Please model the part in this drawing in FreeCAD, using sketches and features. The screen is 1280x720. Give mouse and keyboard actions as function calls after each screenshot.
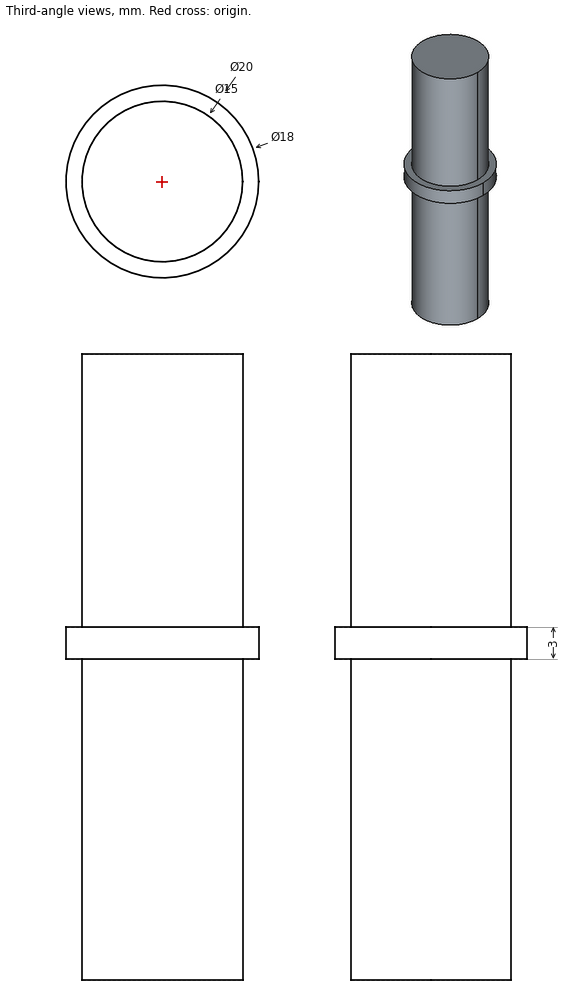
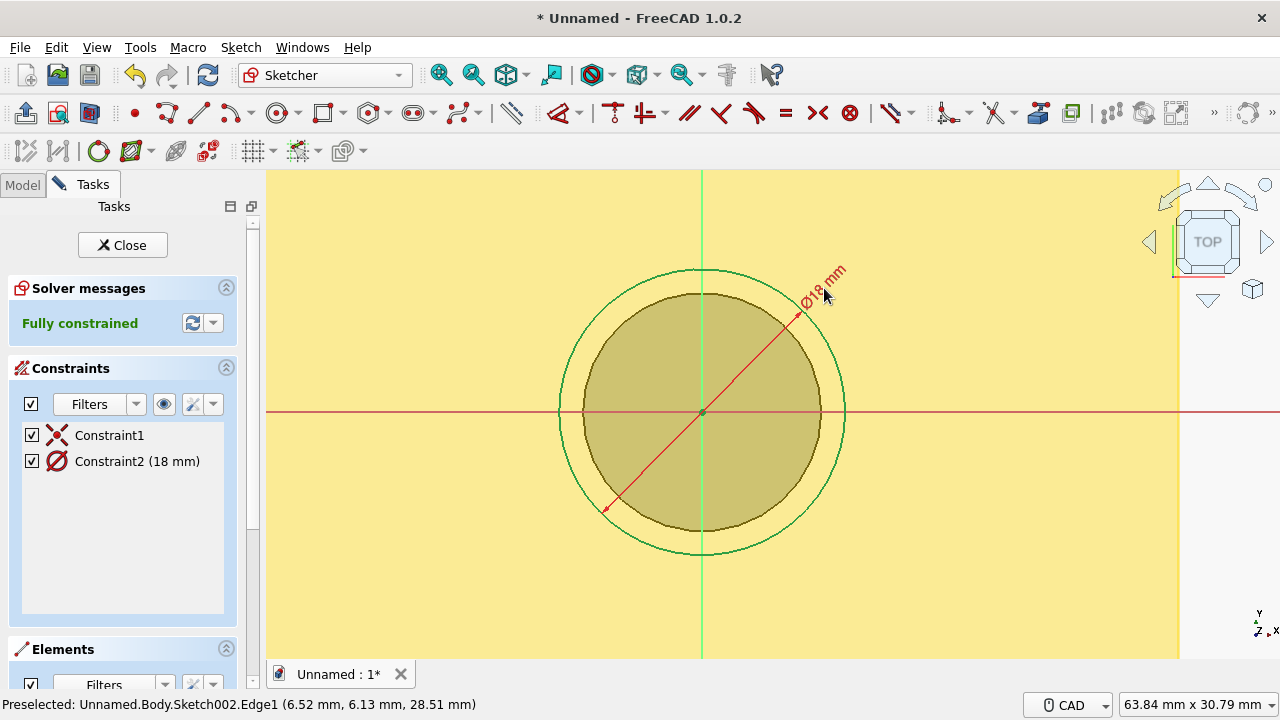
click(123, 245)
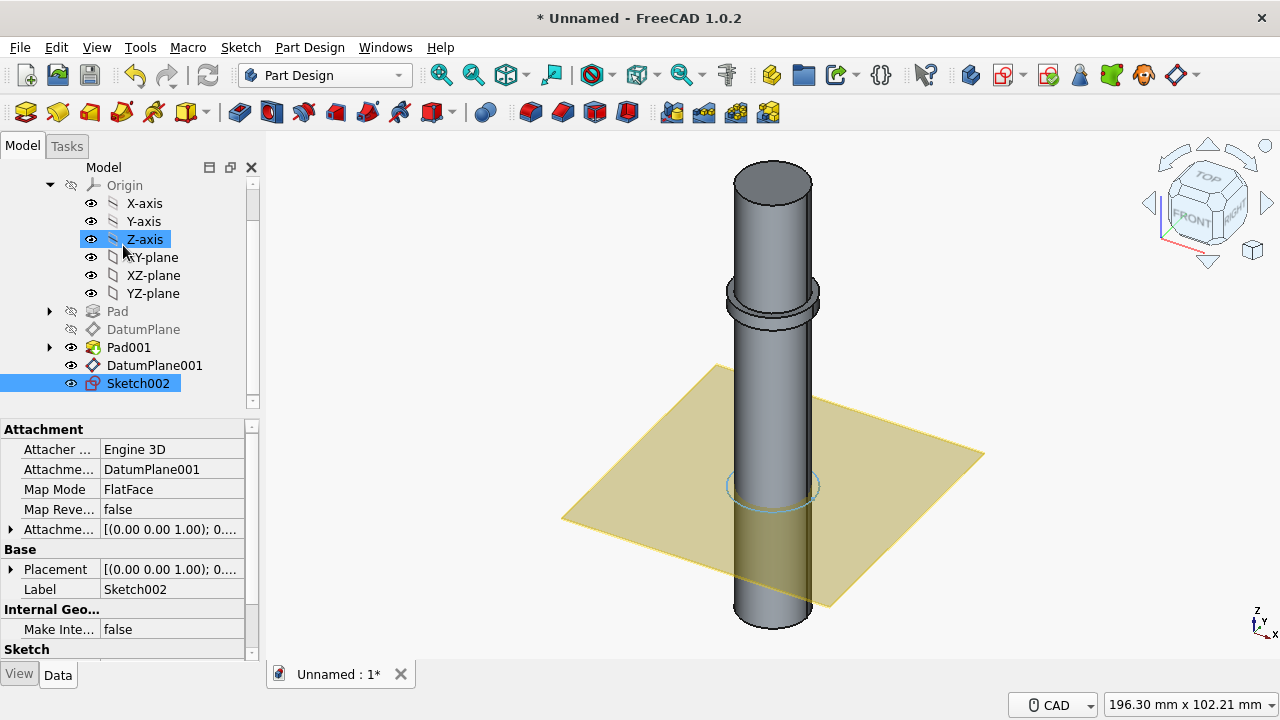
click(26, 112)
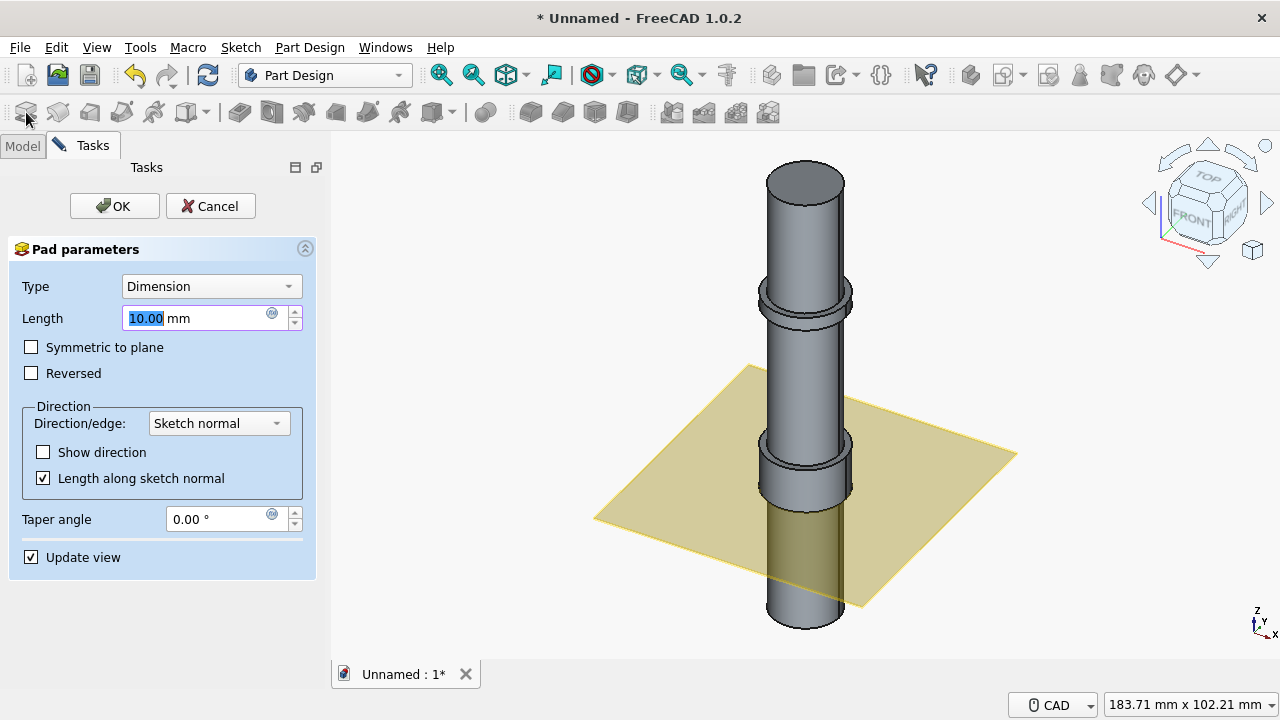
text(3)
key(Tab)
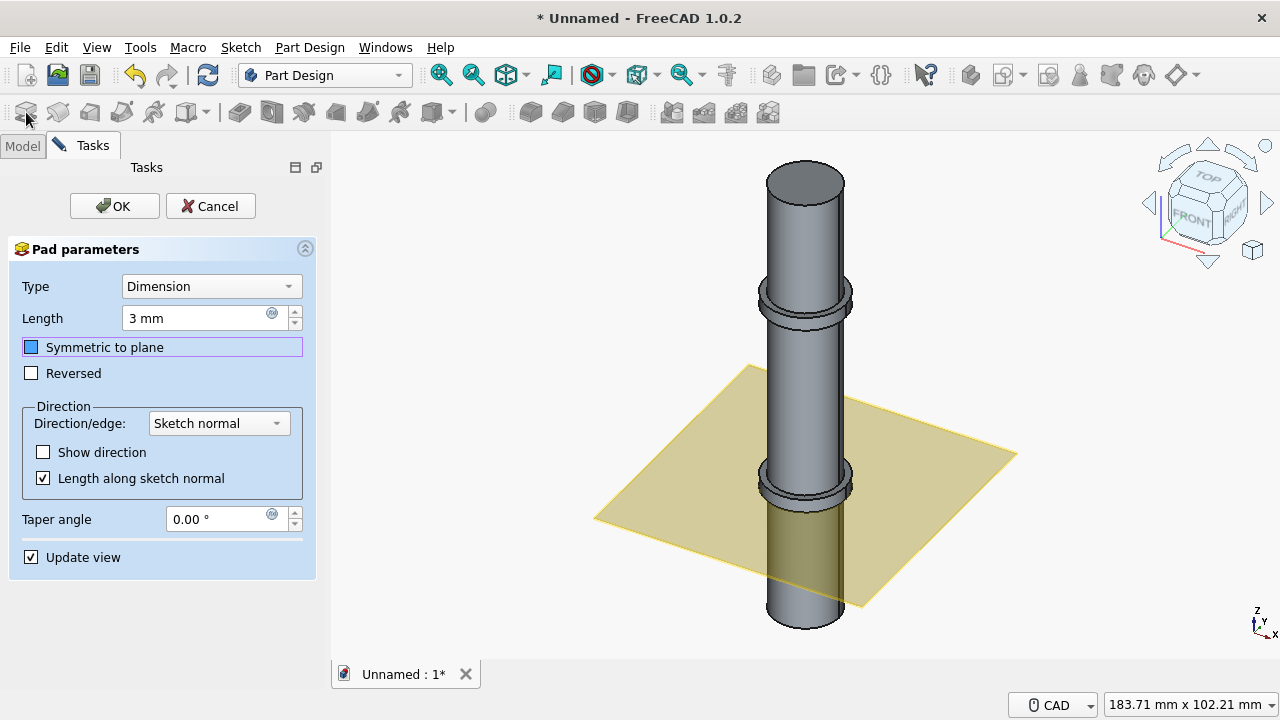
click(30, 373)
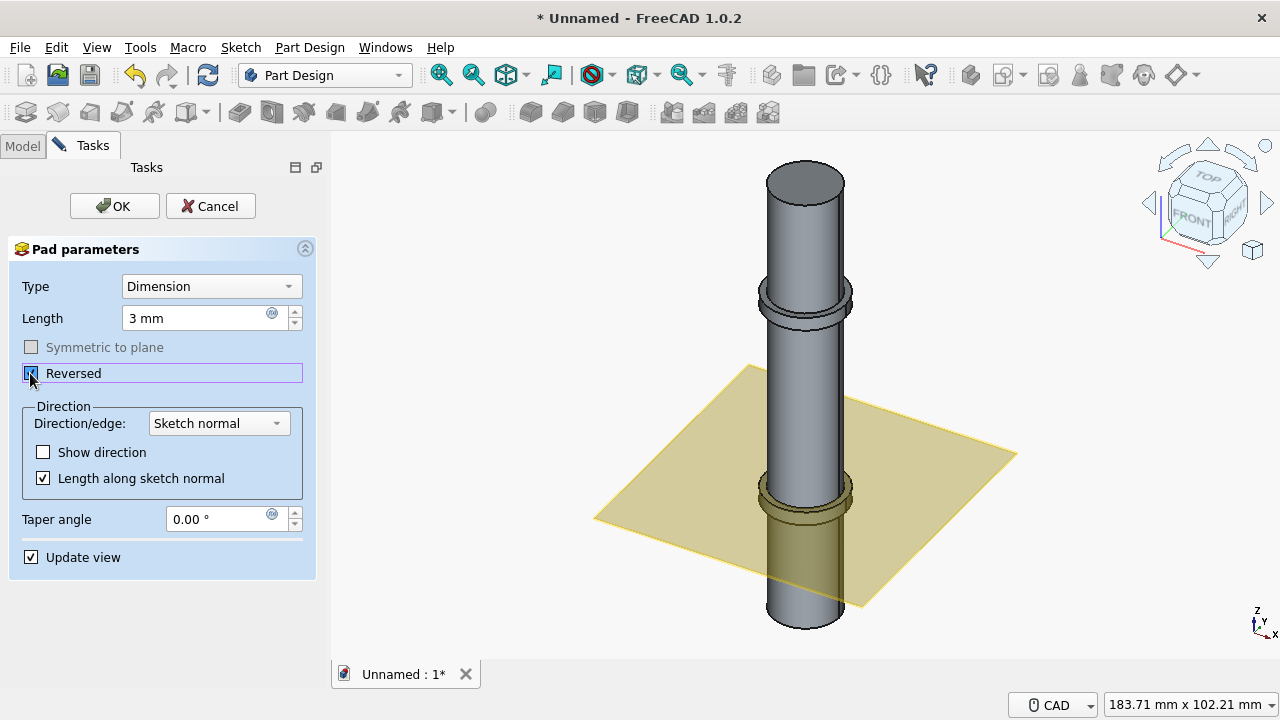
click(115, 206)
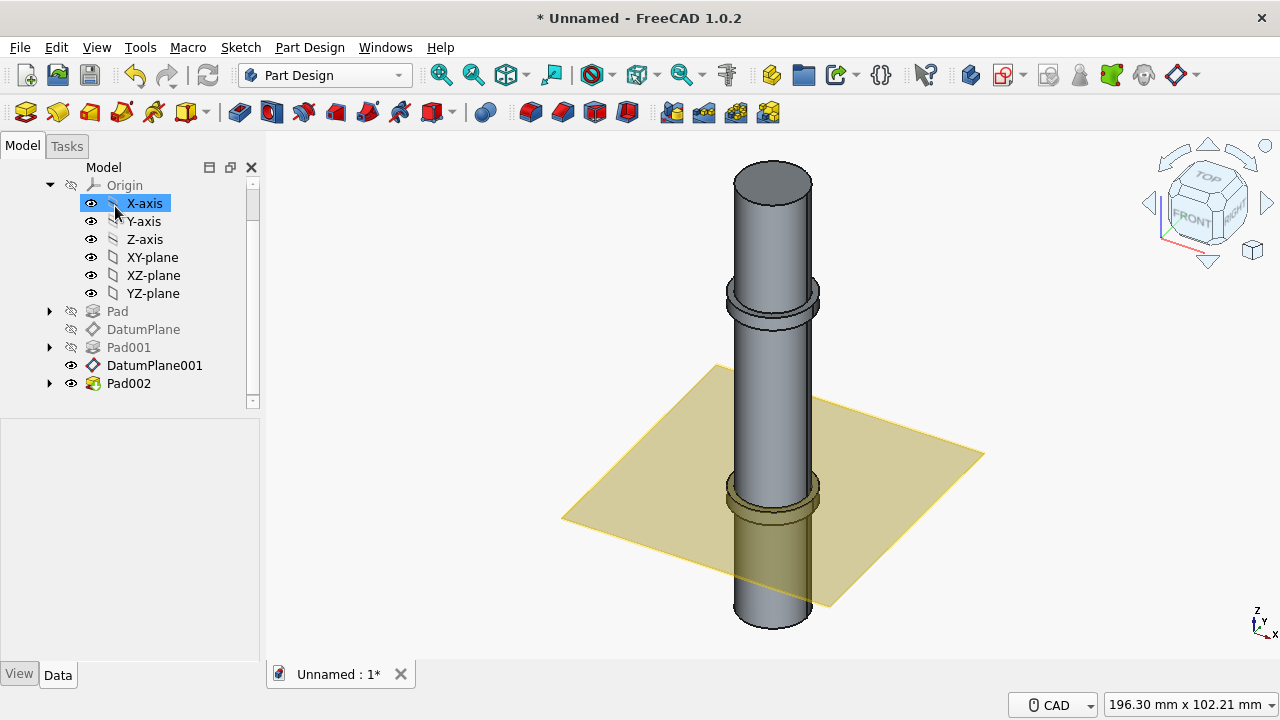
click(116, 365)
key(space)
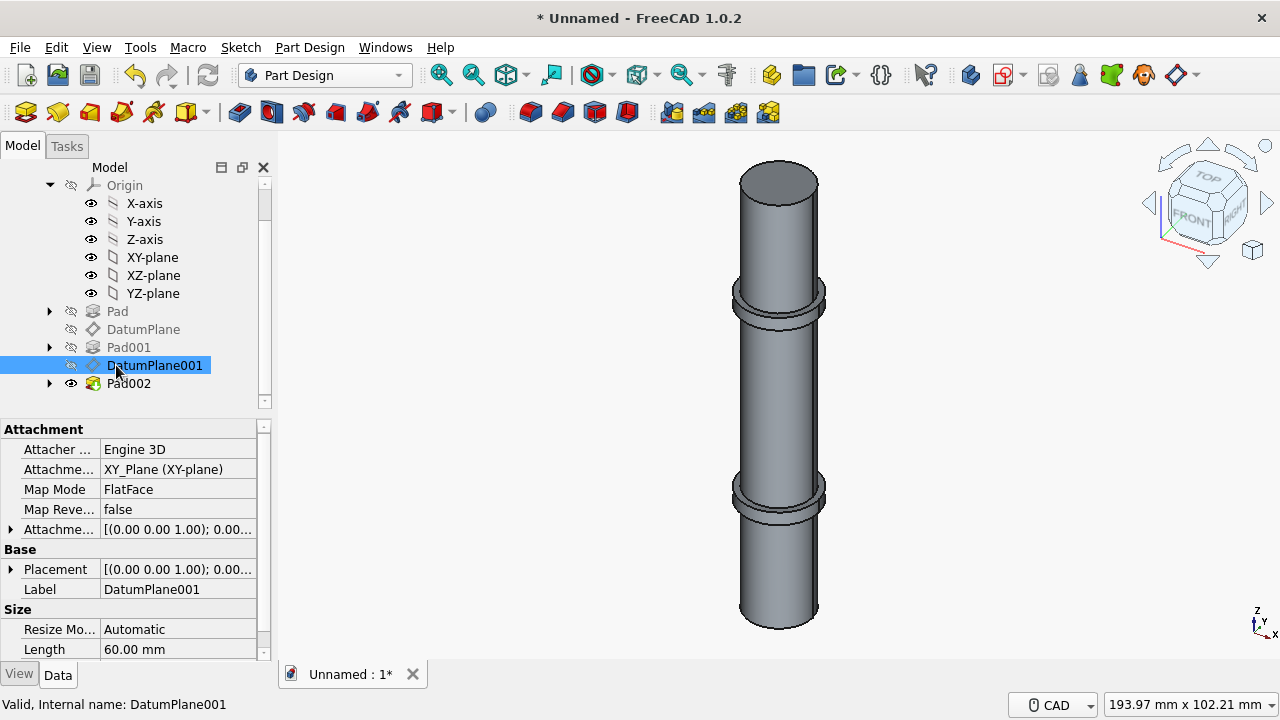
click(136, 257)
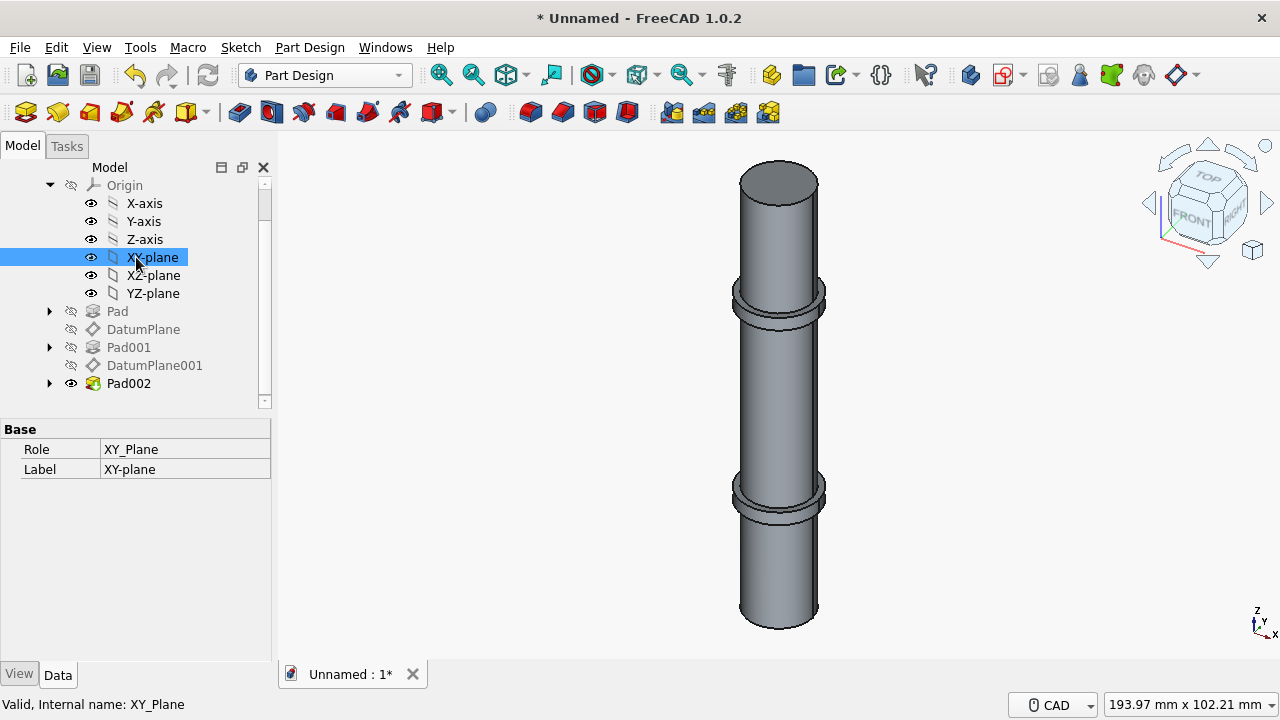
click(1176, 76)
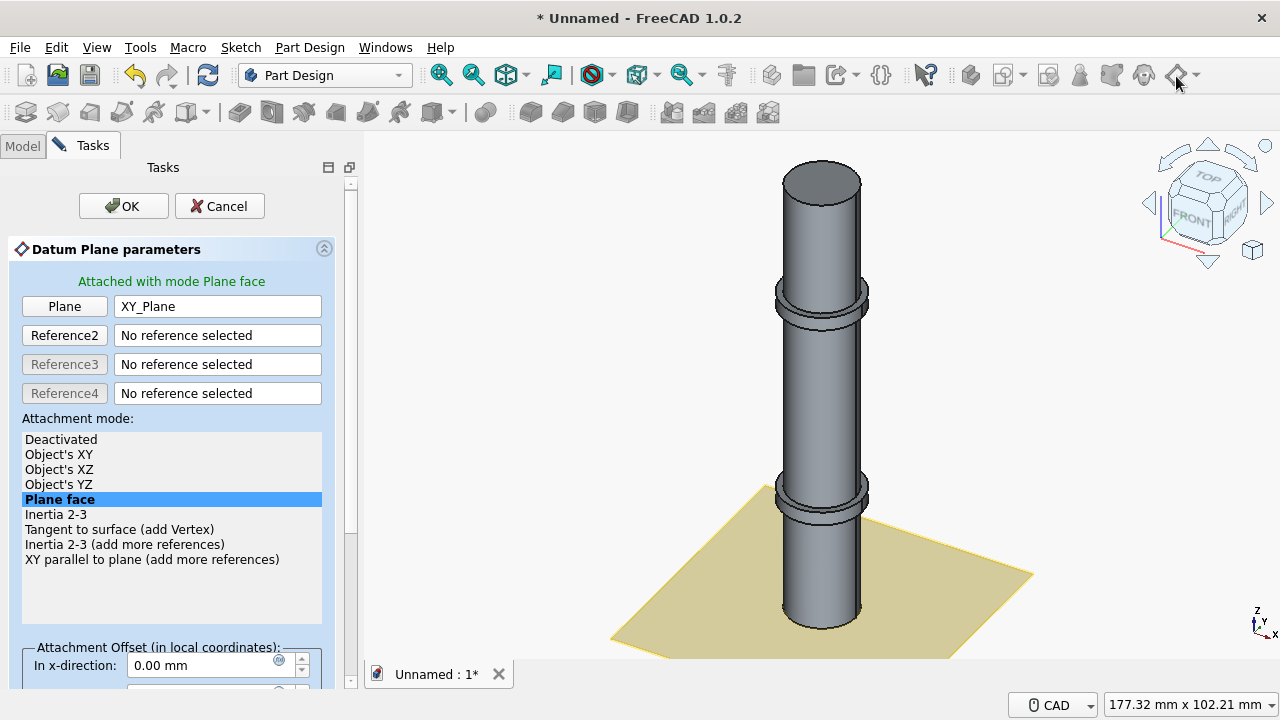
scroll(351, 432, down, 2)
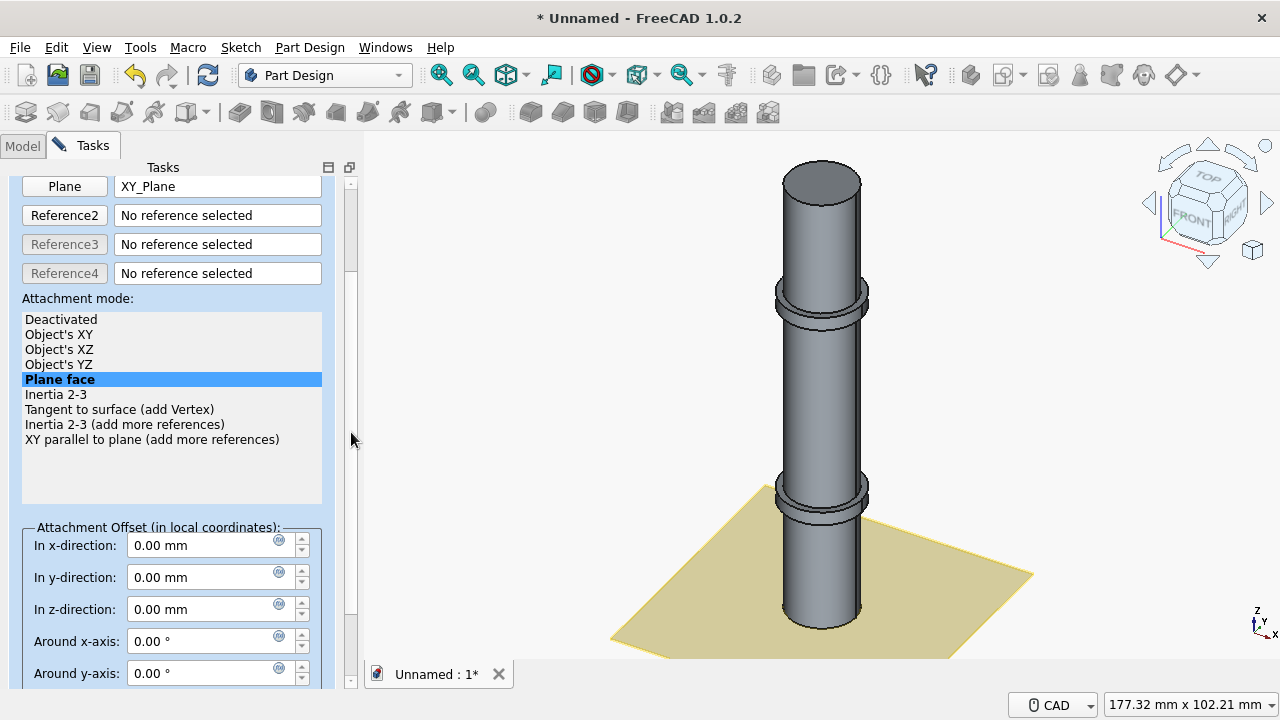
triple_click(210, 609)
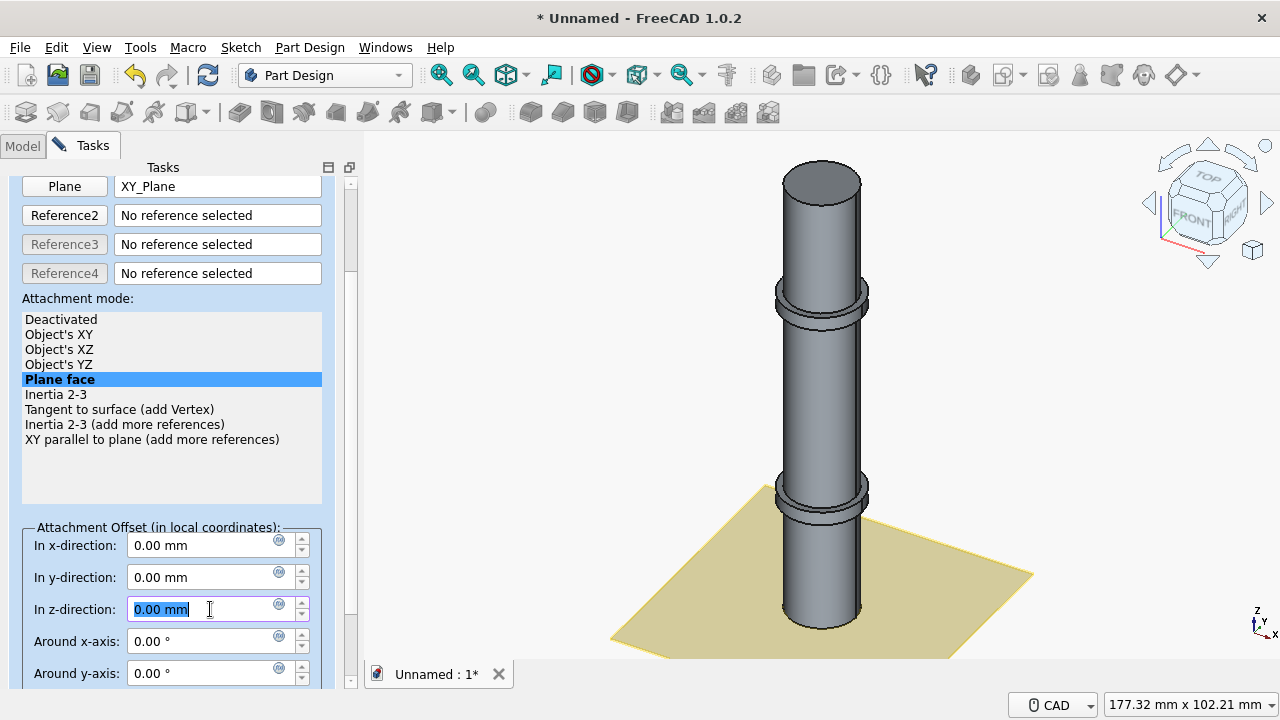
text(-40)
key(Tab)